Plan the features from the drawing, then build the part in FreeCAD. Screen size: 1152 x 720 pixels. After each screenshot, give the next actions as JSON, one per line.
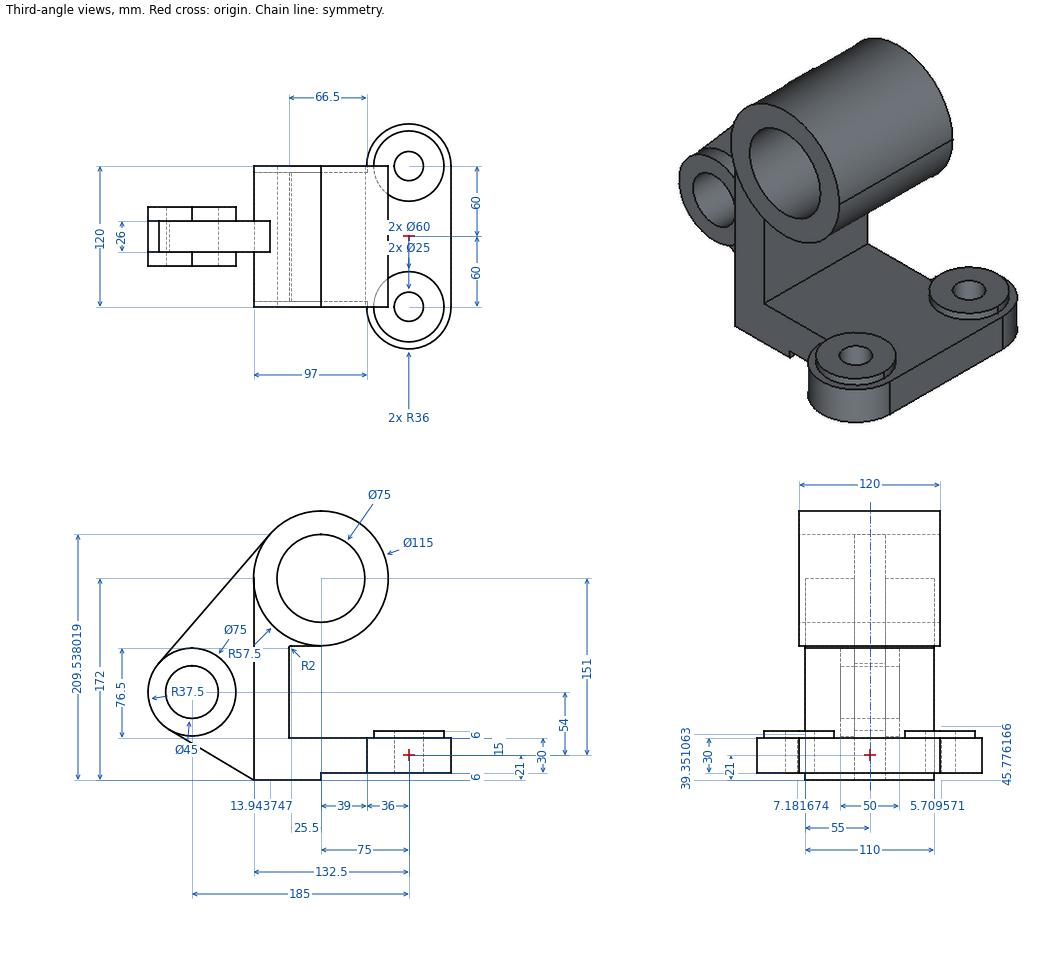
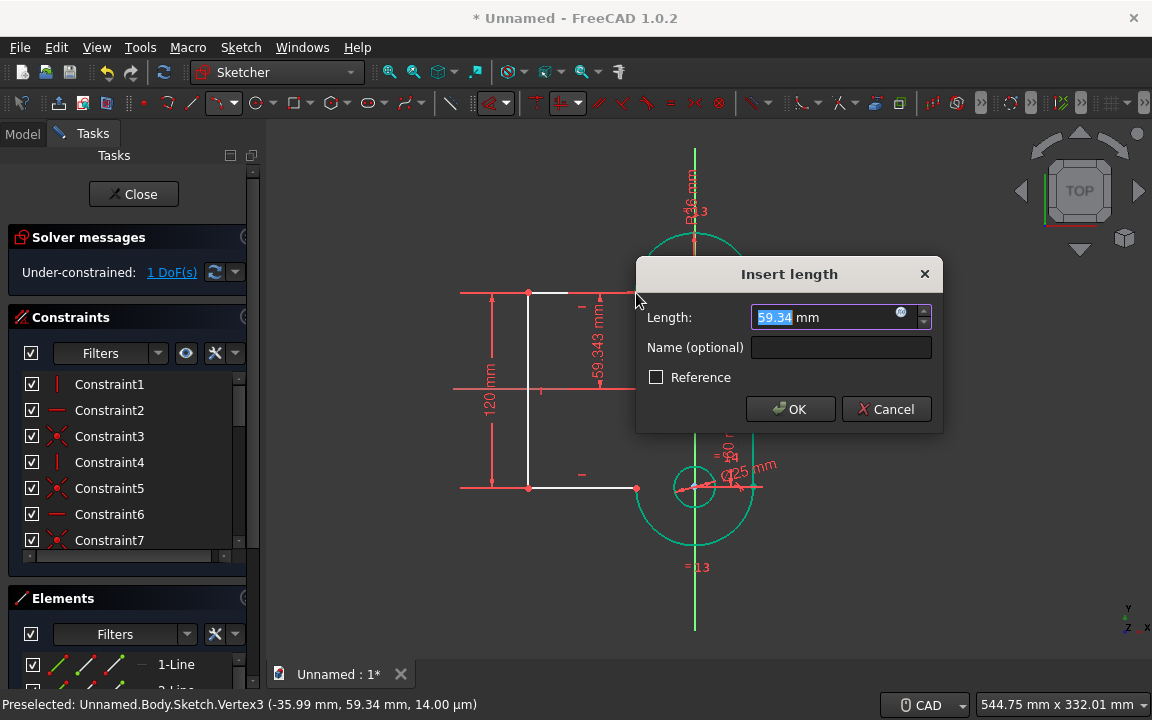
{"action": "type", "text": "60"}
{"action": "key", "text": "Return"}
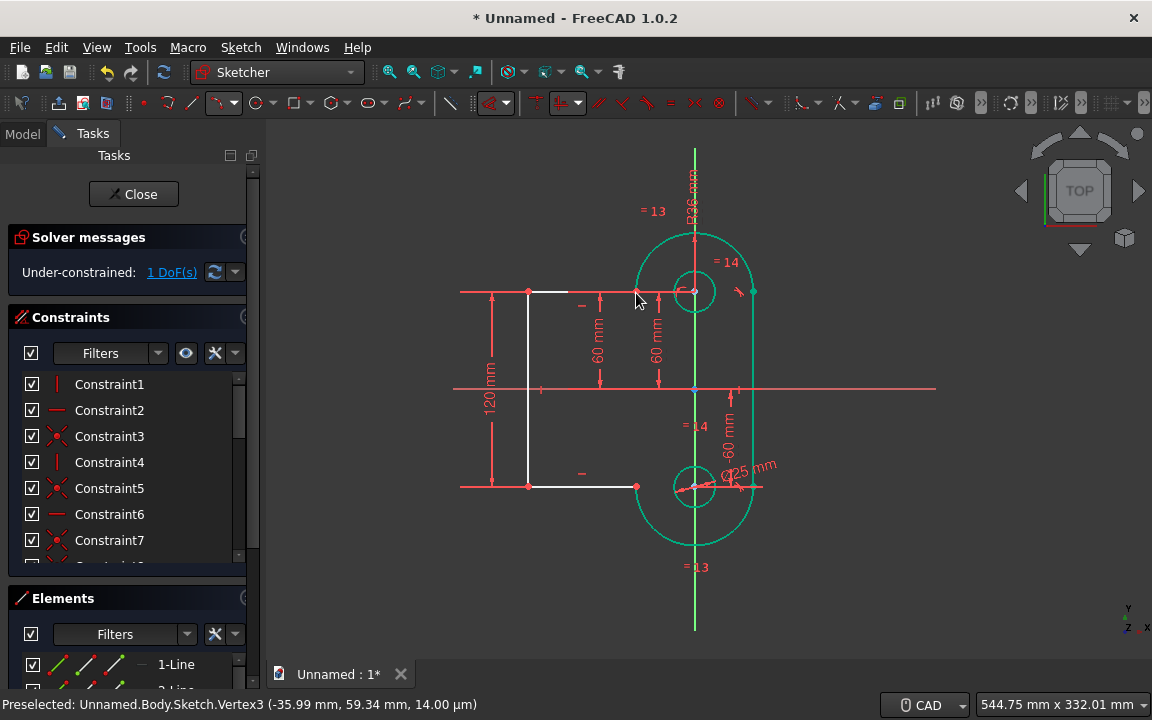
{"action": "left_click", "coordinate": [604, 292]}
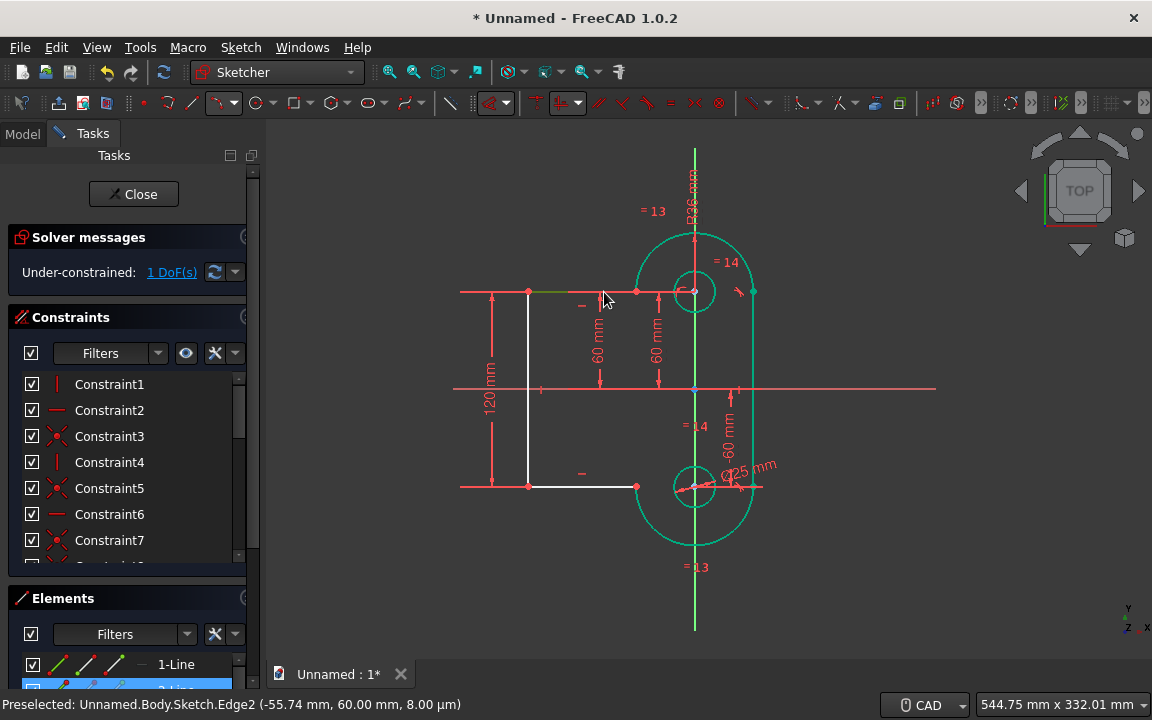
{"action": "key", "text": "l"}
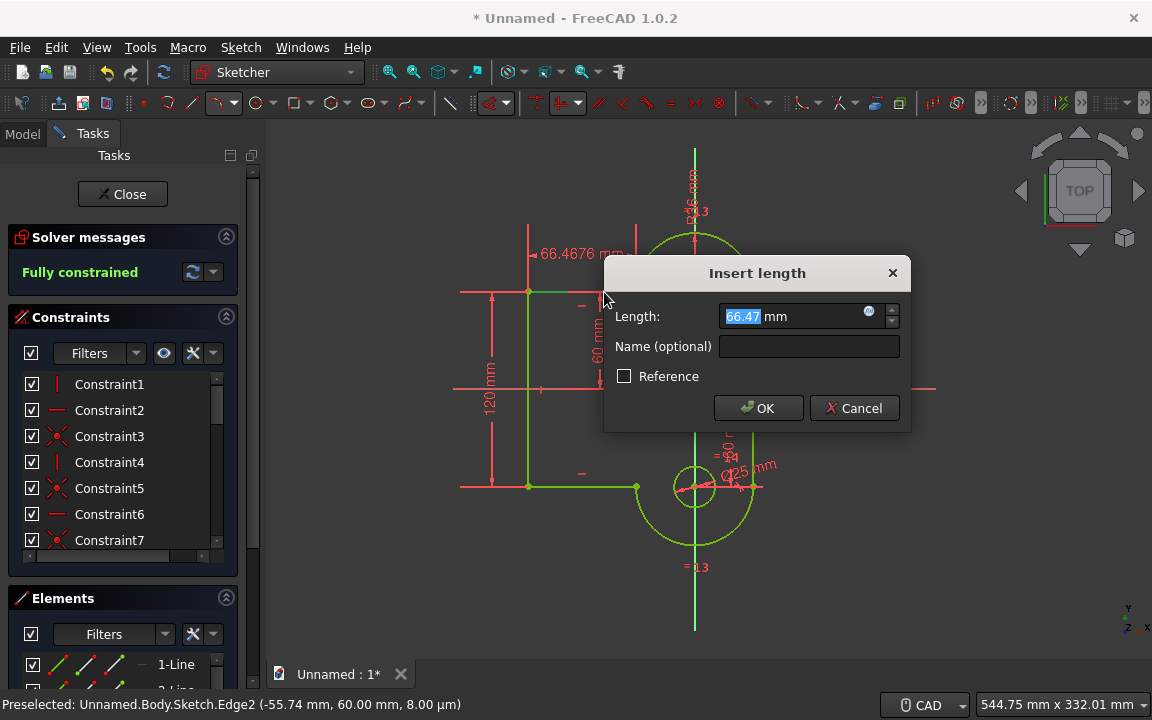
{"action": "type", "text": "66.5"}
{"action": "key", "text": "Return"}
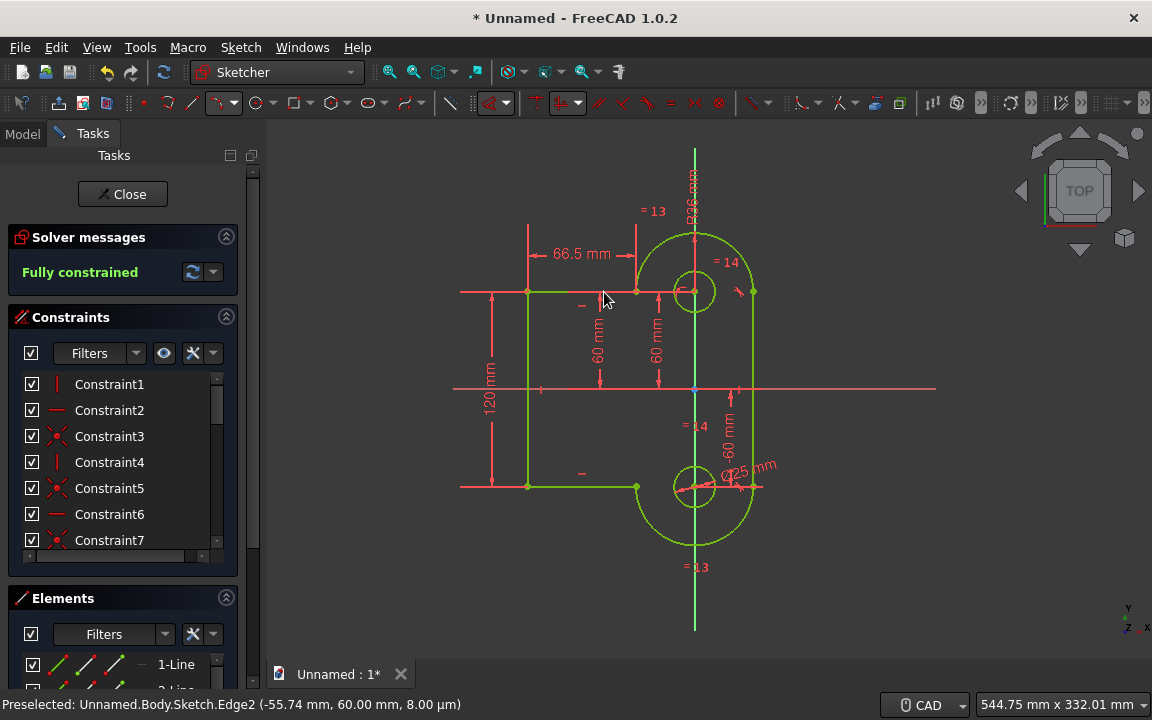
{"action": "left_click", "coordinate": [123, 194]}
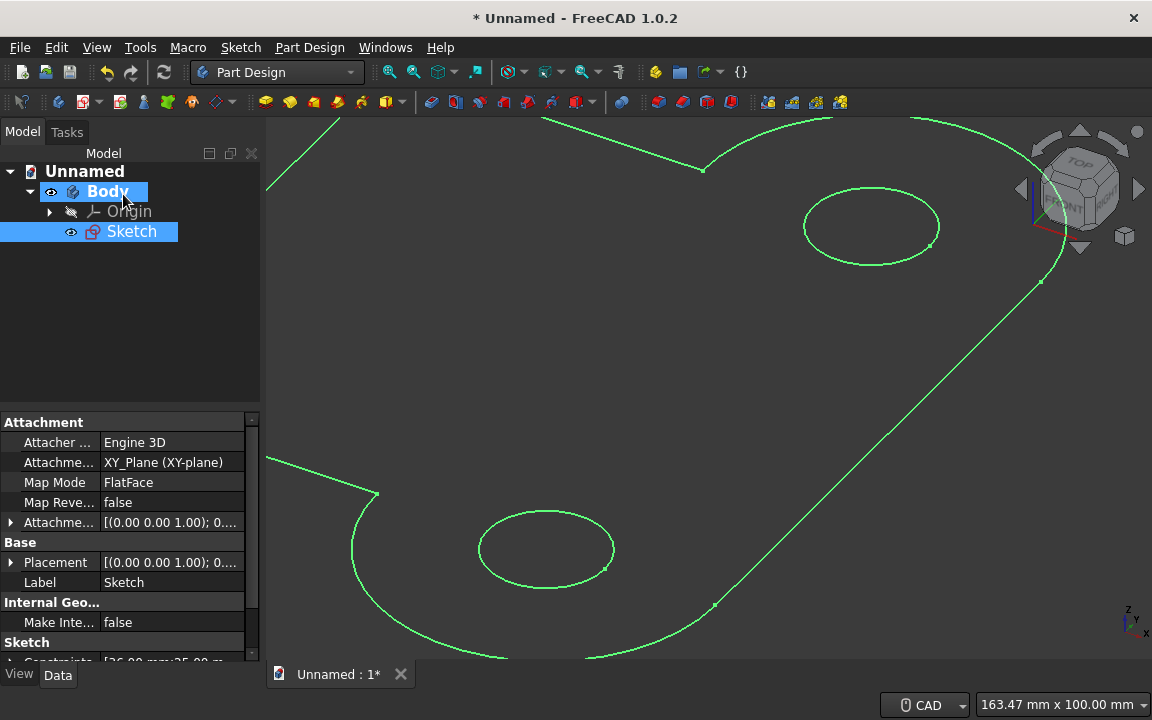
{"action": "left_click", "coordinate": [266, 102]}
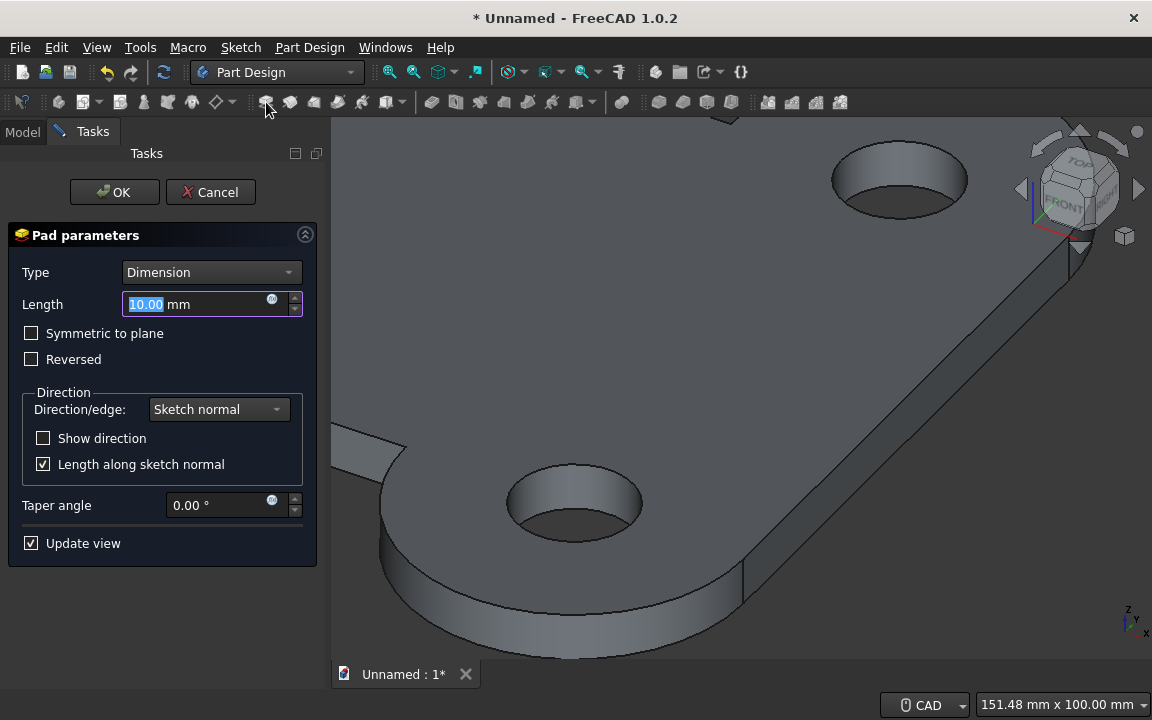
{"action": "type", "text": "30"}
{"action": "key", "text": "Tab"}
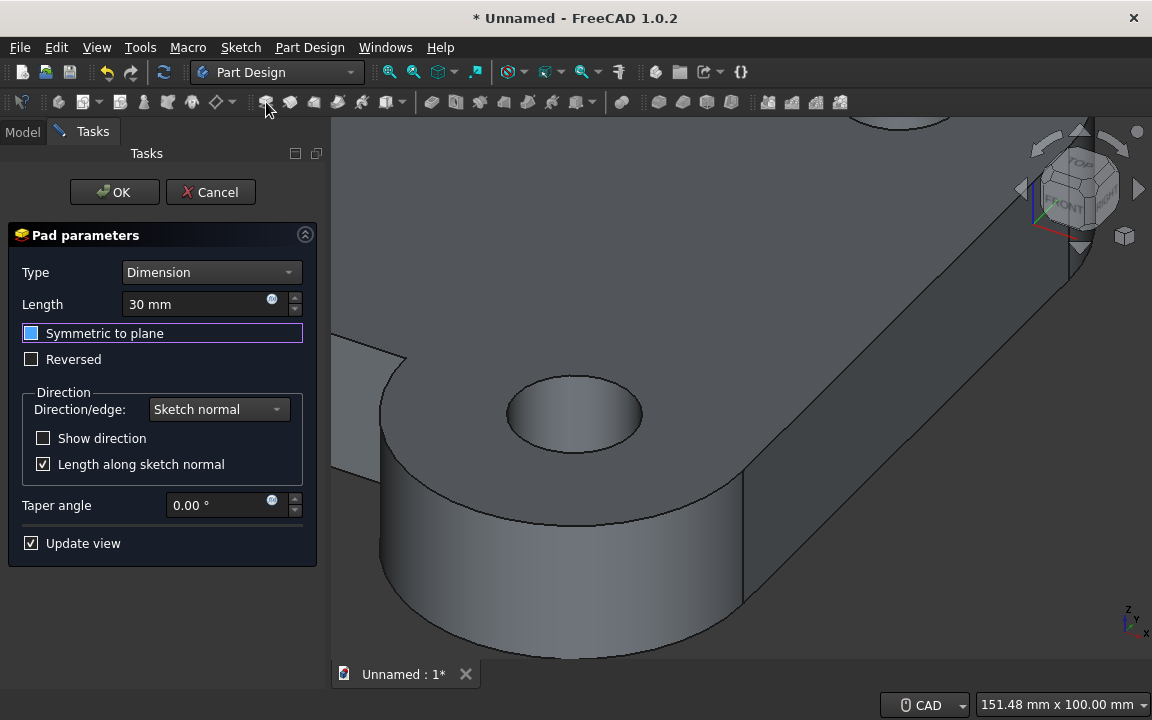
{"action": "left_click", "coordinate": [30, 333]}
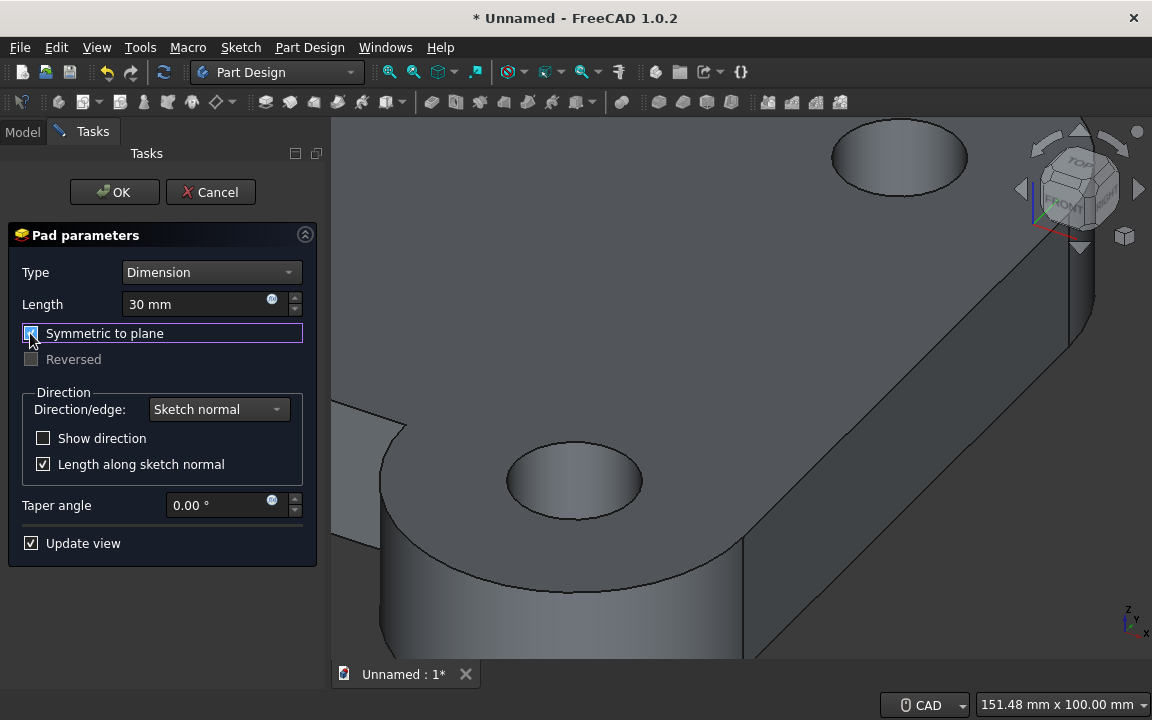
{"action": "left_click", "coordinate": [115, 192]}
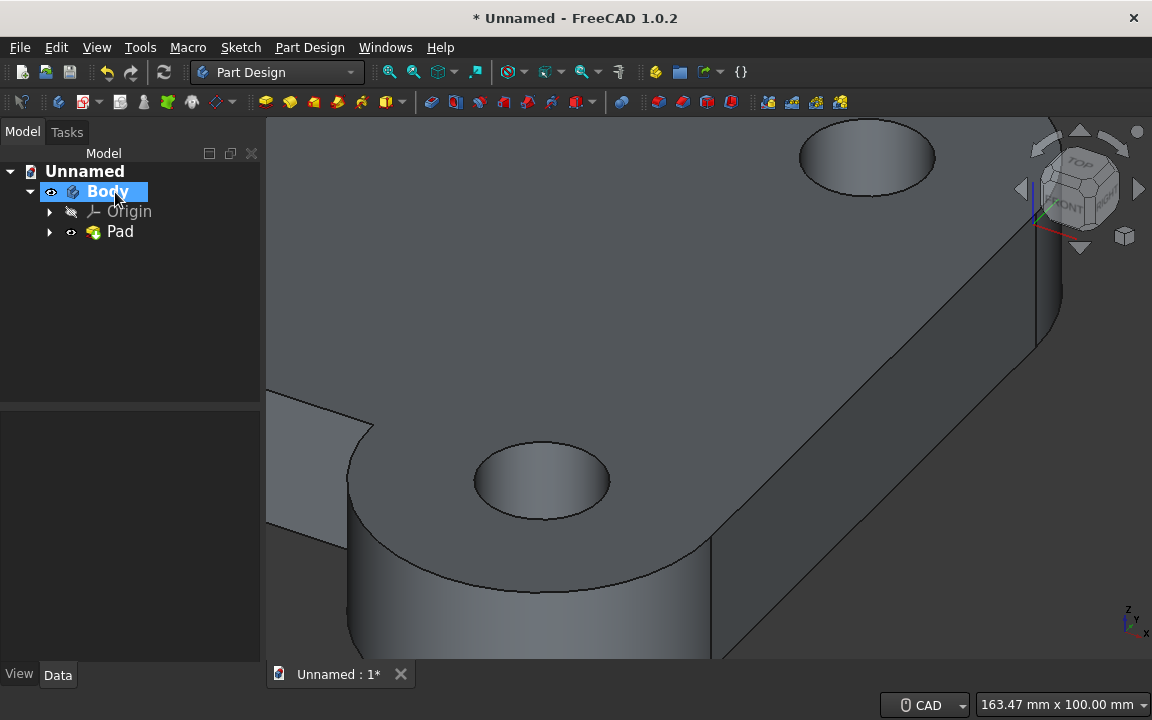
{"action": "key", "text": "v f"}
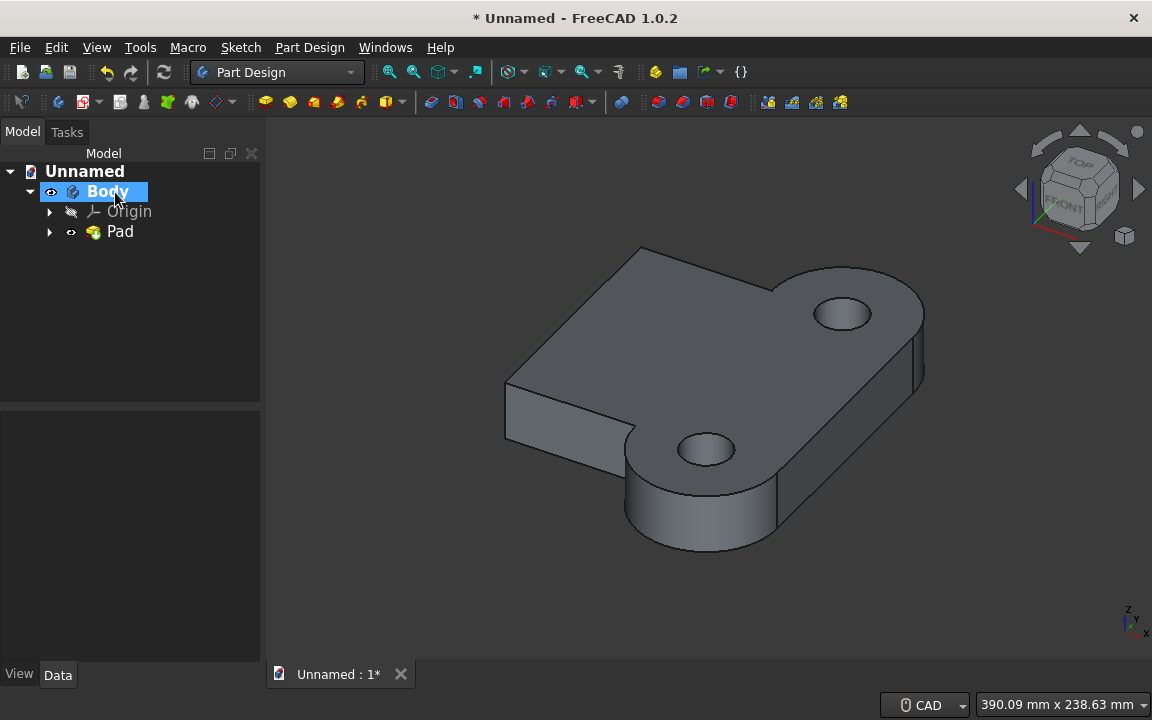
{"action": "left_click", "coordinate": [709, 359]}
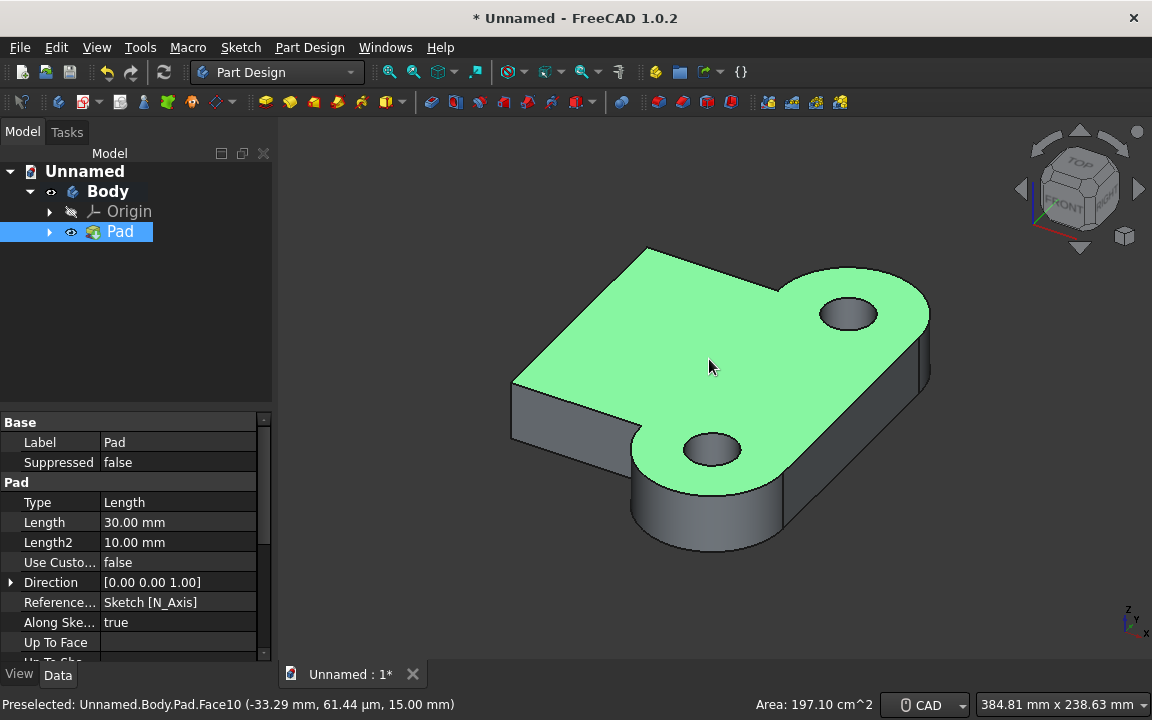
{"action": "left_click", "coordinate": [84, 102]}